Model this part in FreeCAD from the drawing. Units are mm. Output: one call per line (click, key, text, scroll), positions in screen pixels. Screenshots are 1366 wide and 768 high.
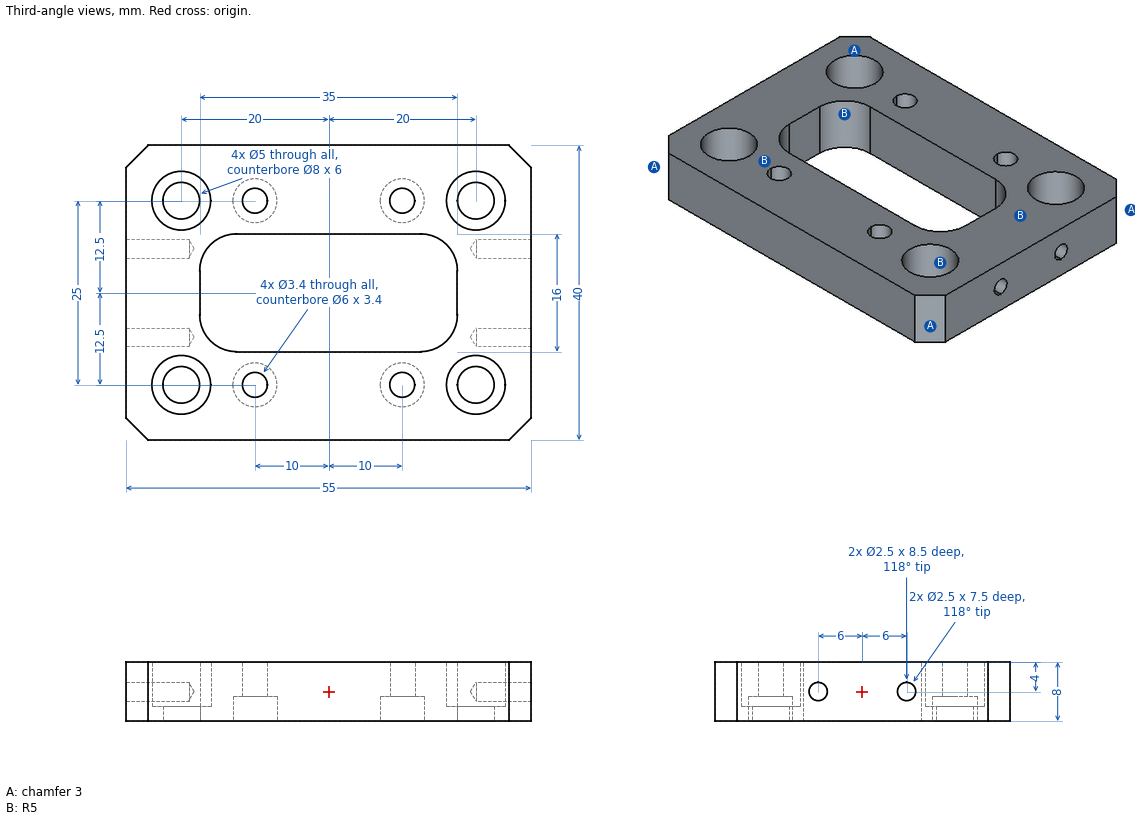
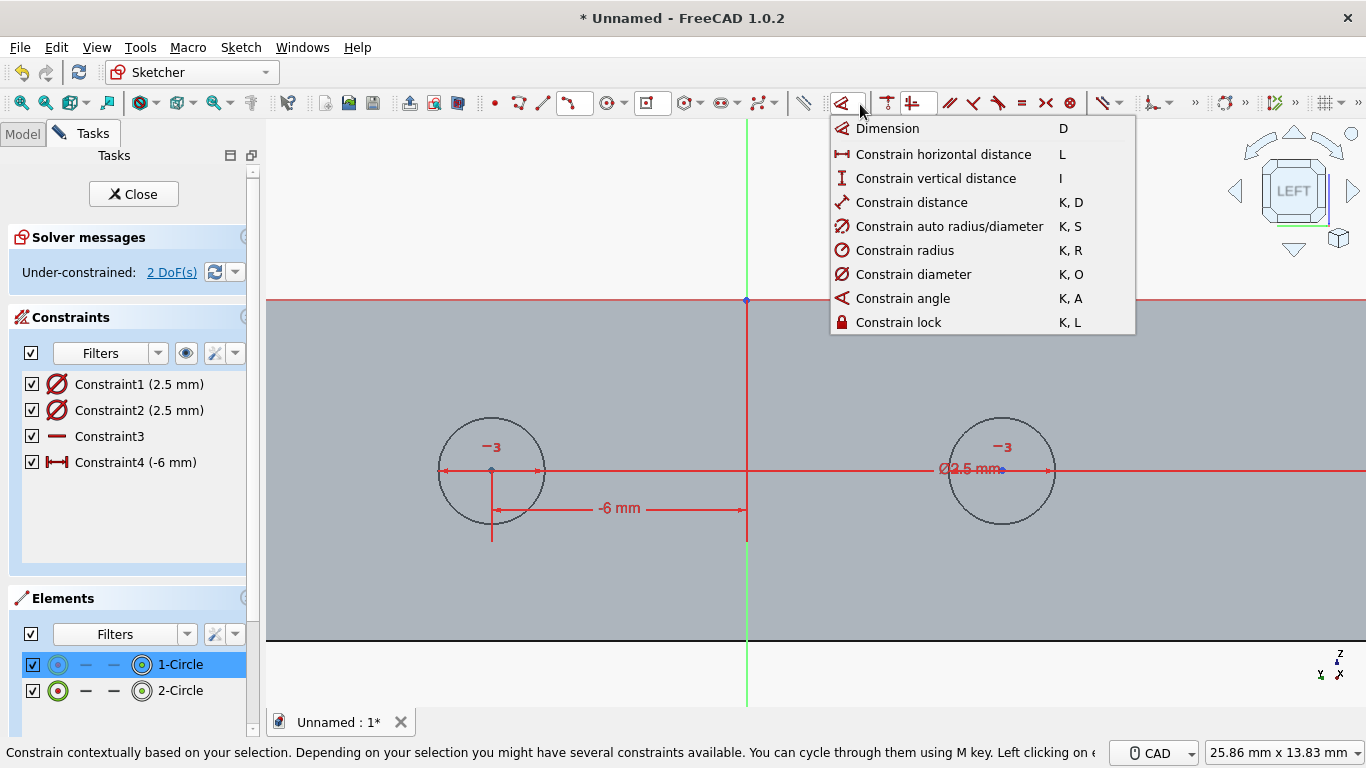
click(983, 178)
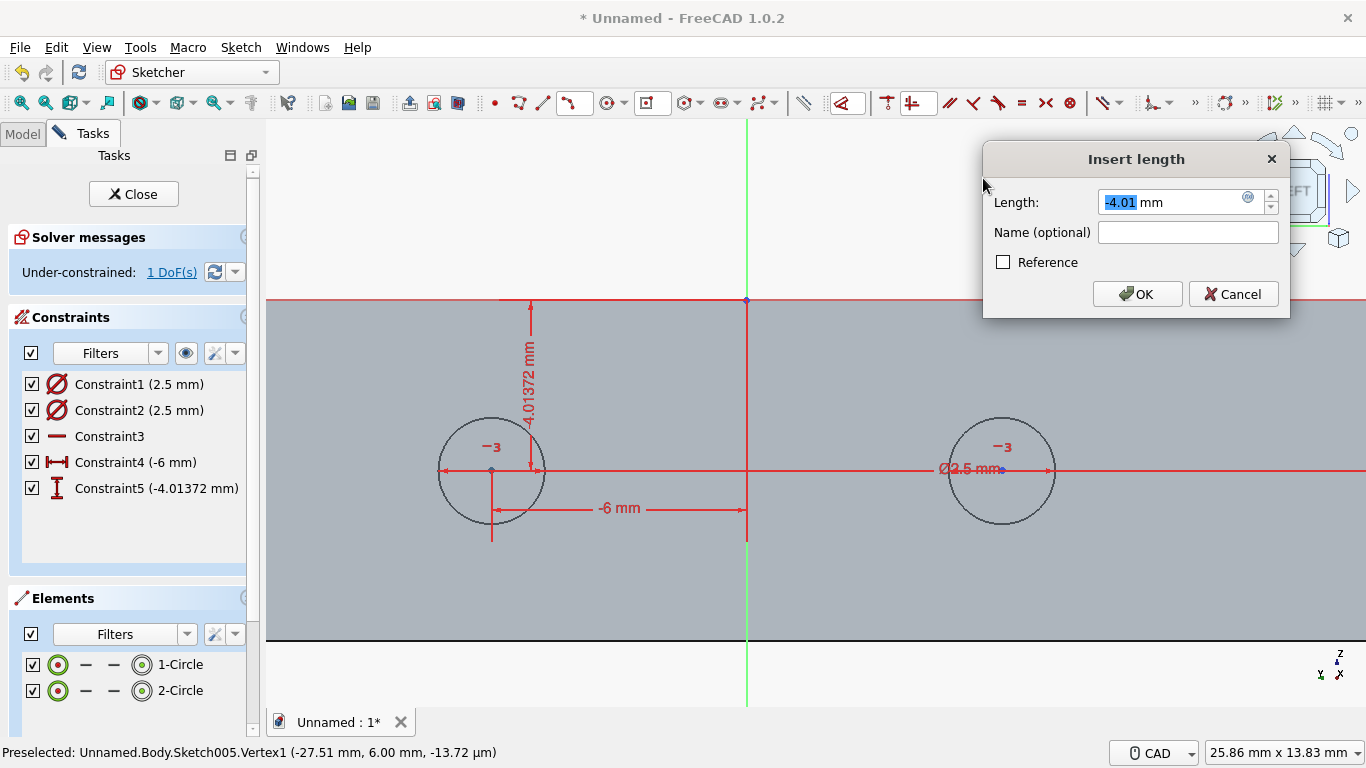
text(-4)
key(Return)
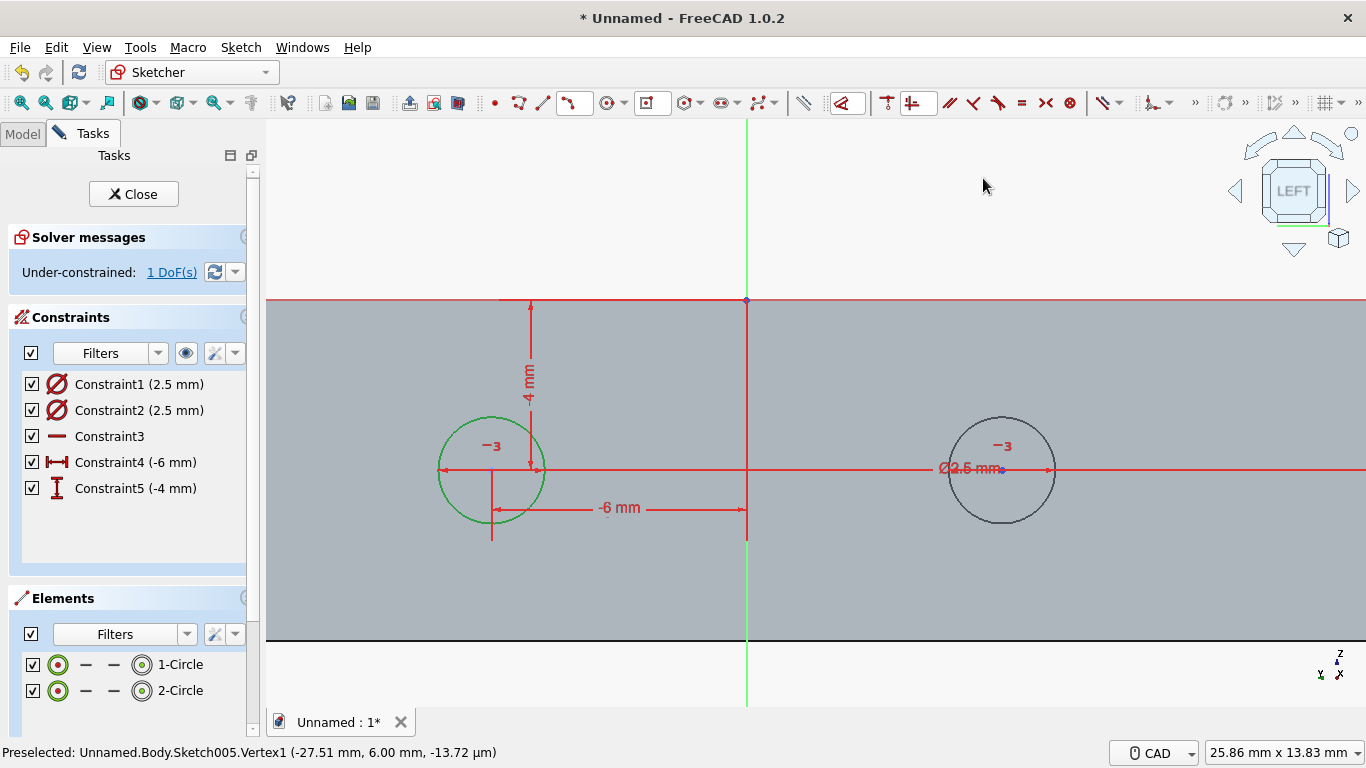
click(1002, 470)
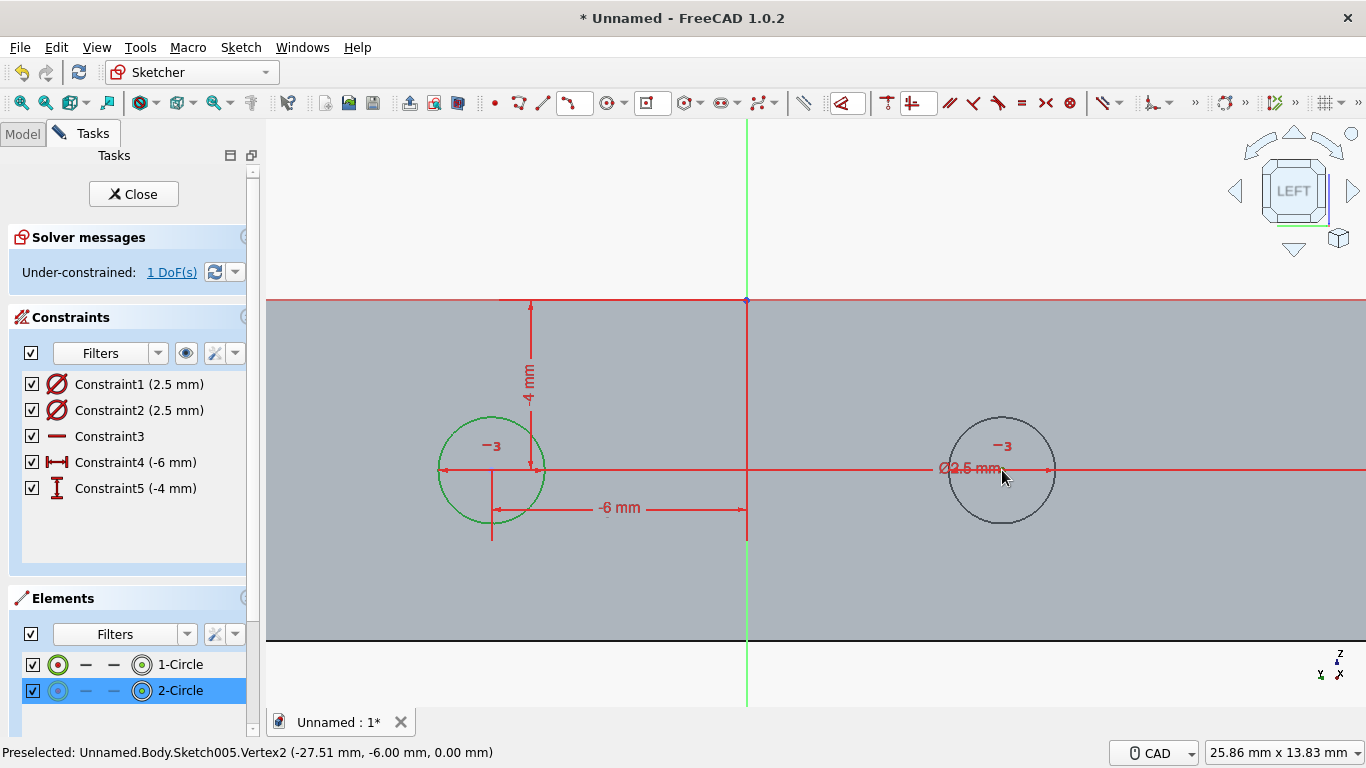
click(860, 104)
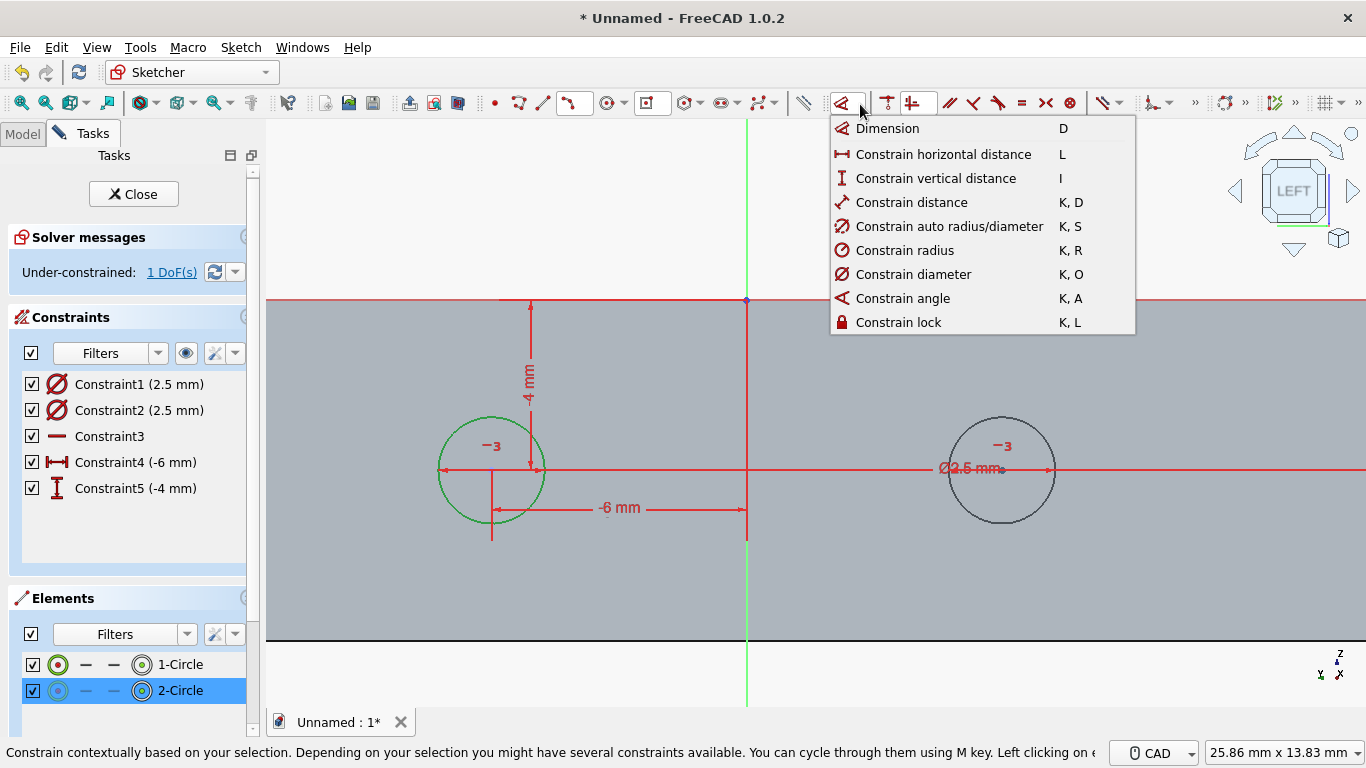
click(983, 154)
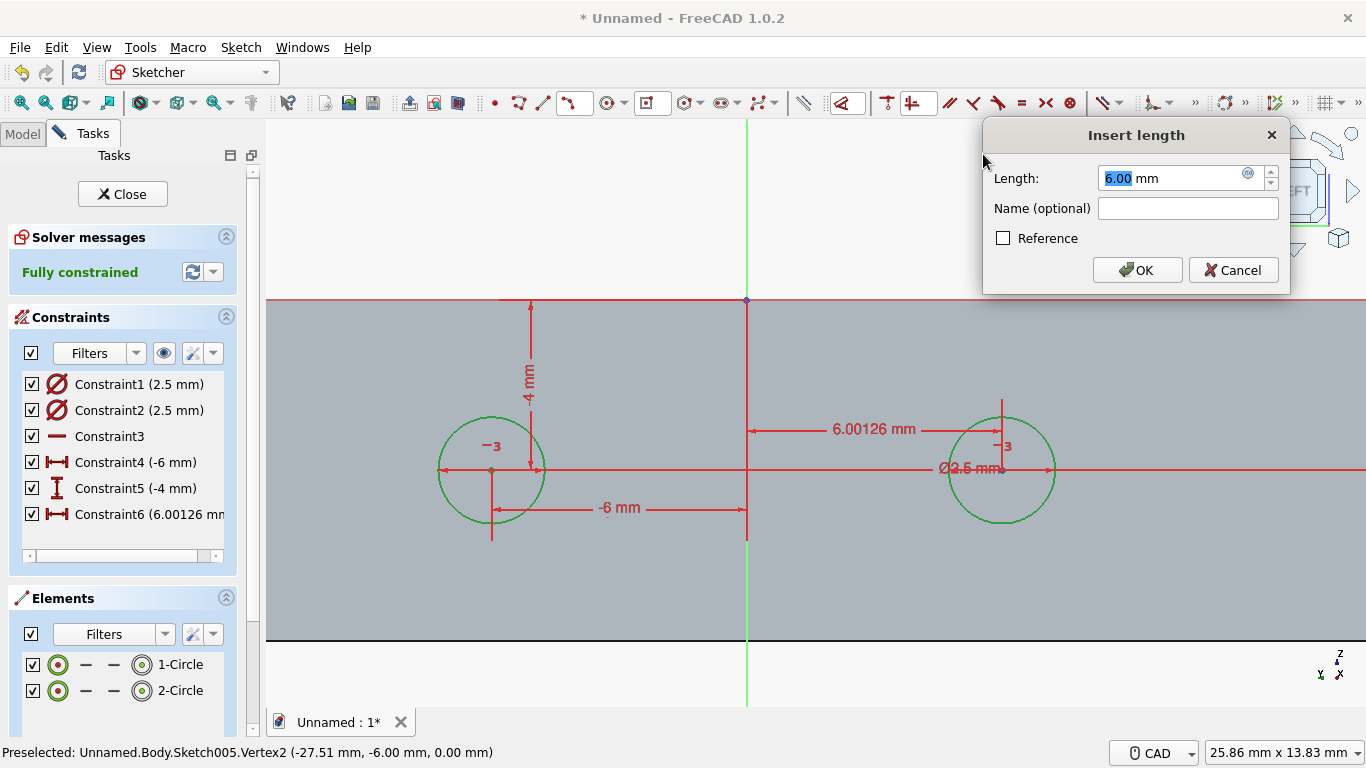
text(6)
key(Return)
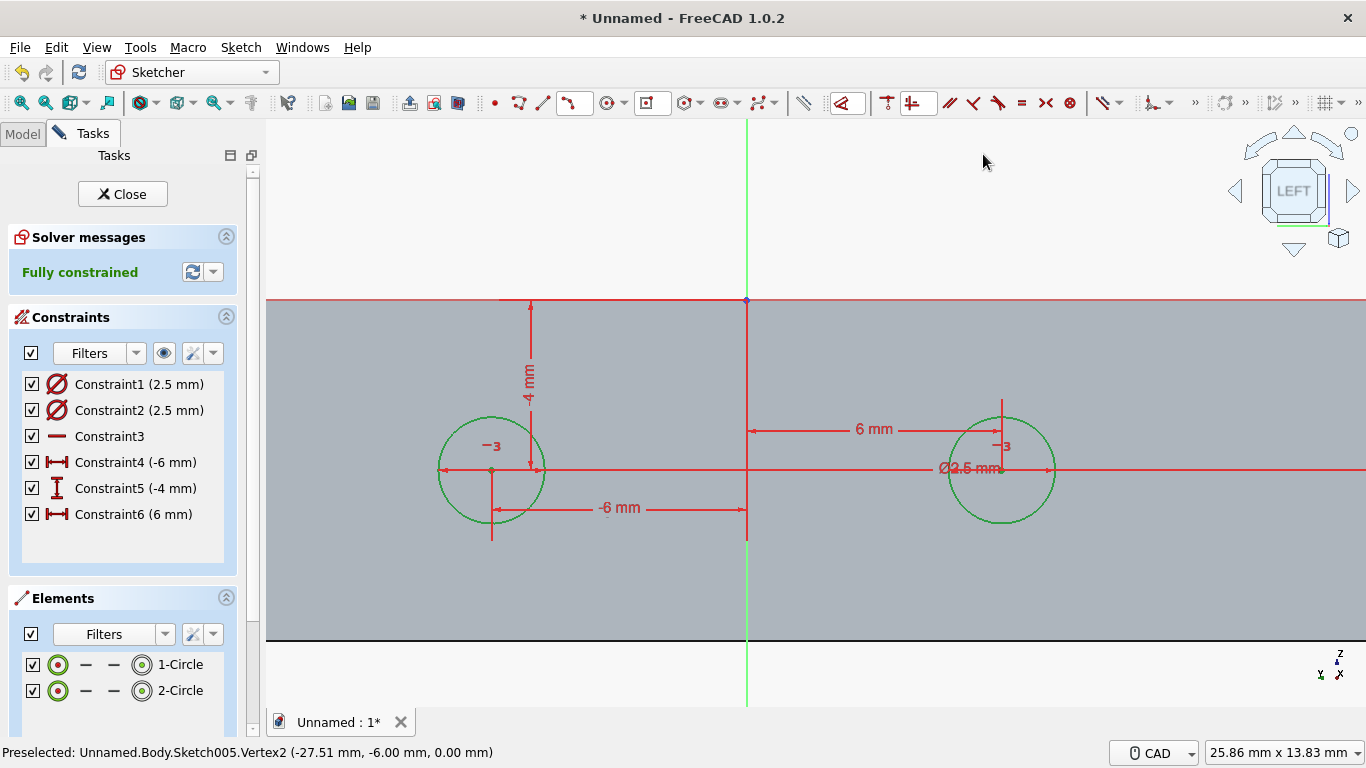
click(123, 194)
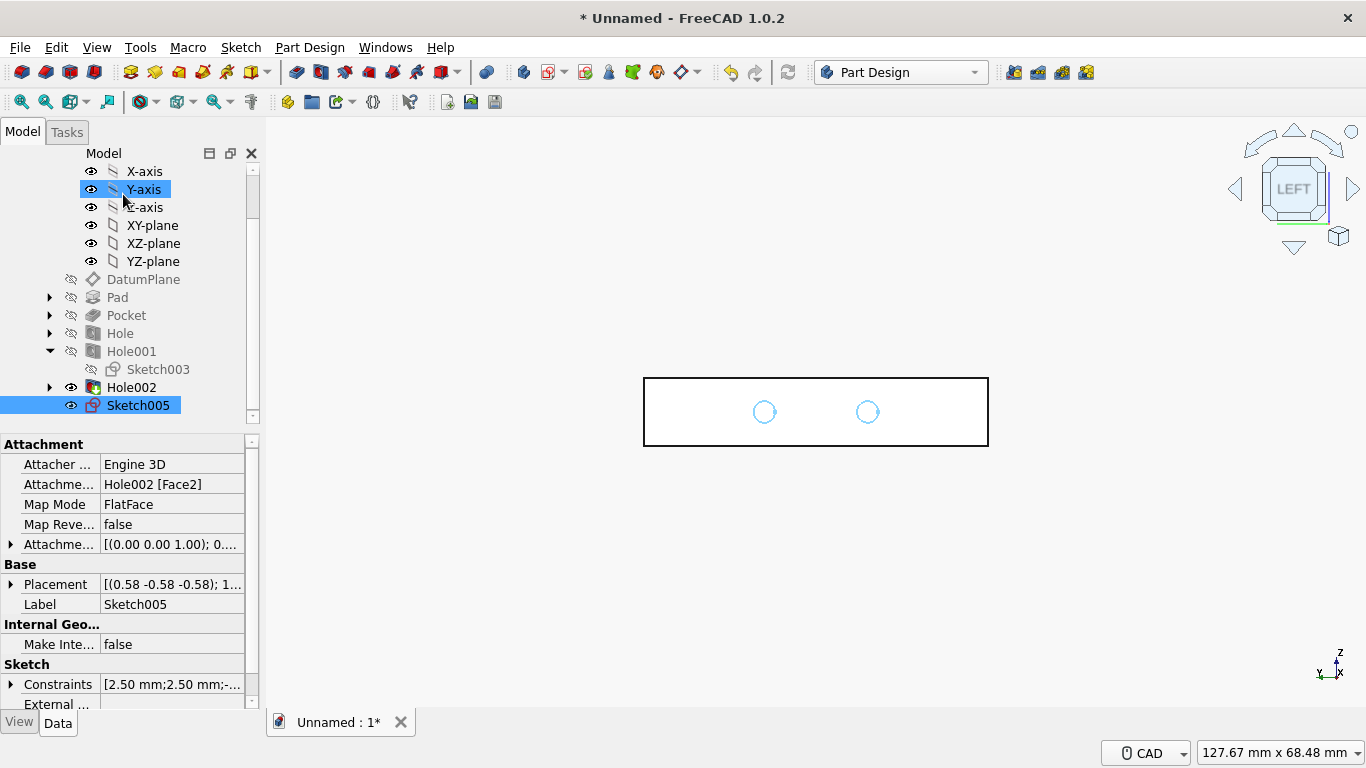
click(322, 72)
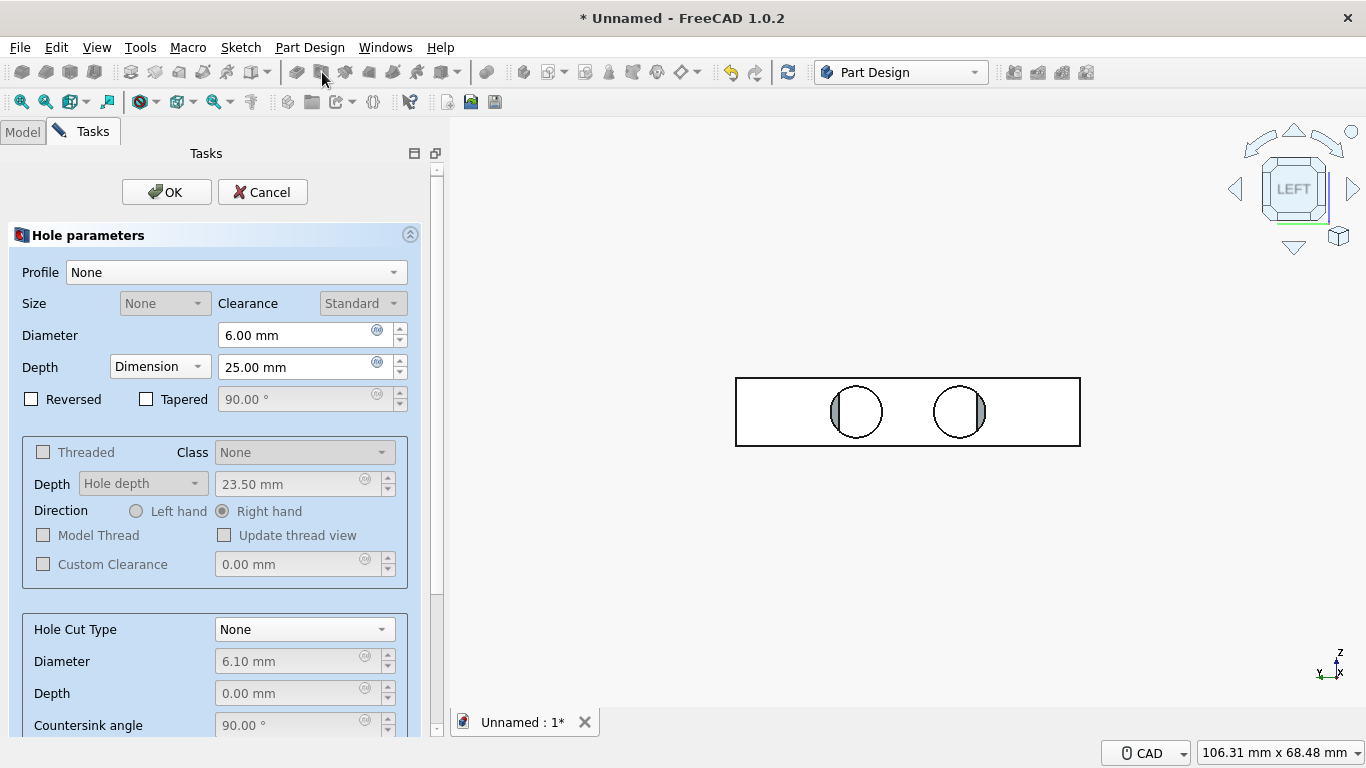
triple_click(305, 335)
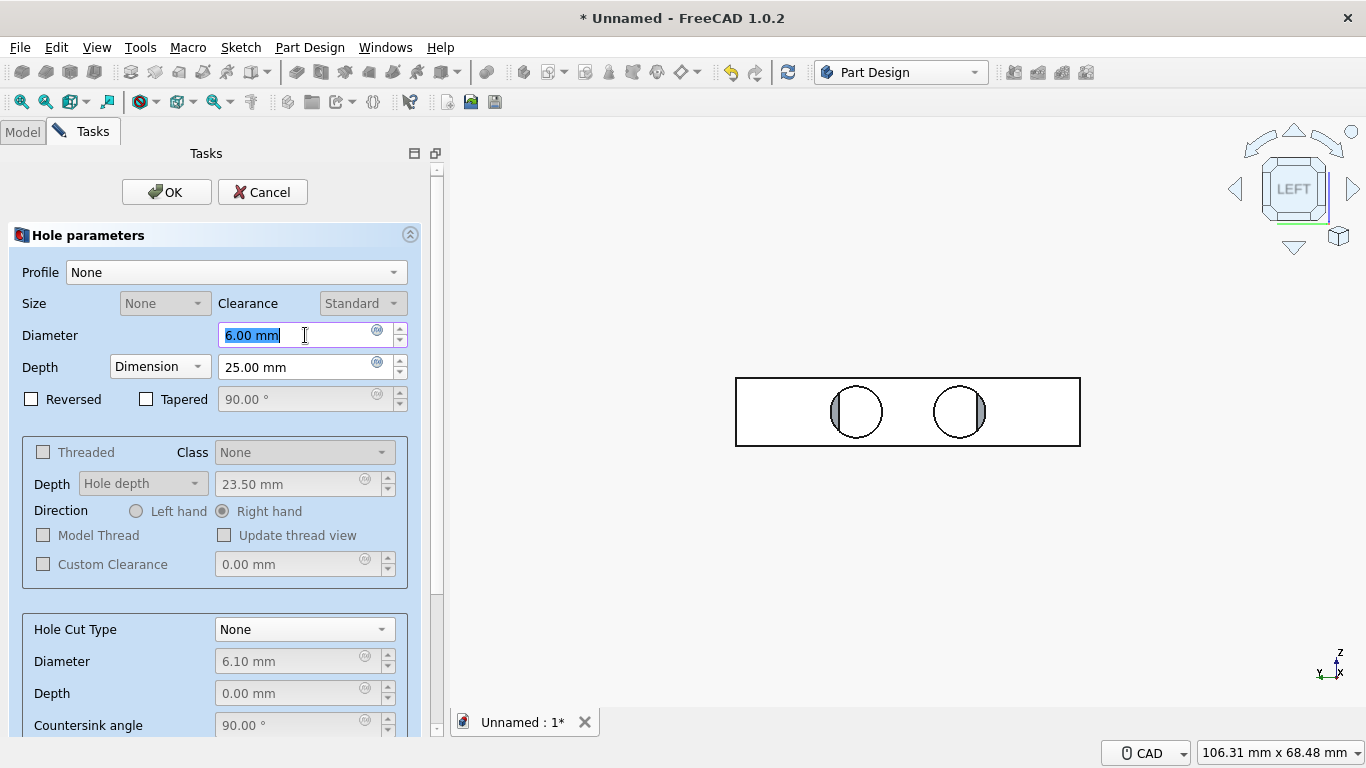
text(2.5)
key(Tab)